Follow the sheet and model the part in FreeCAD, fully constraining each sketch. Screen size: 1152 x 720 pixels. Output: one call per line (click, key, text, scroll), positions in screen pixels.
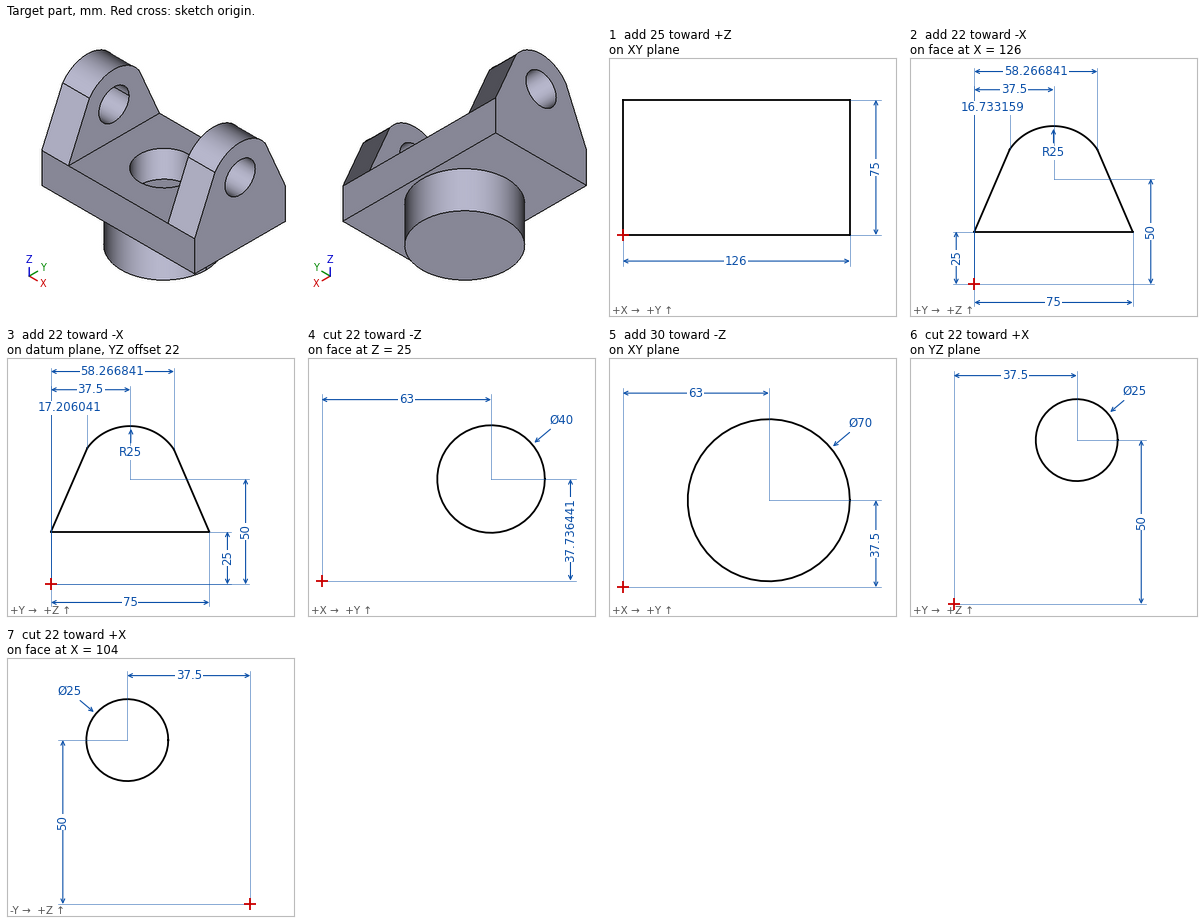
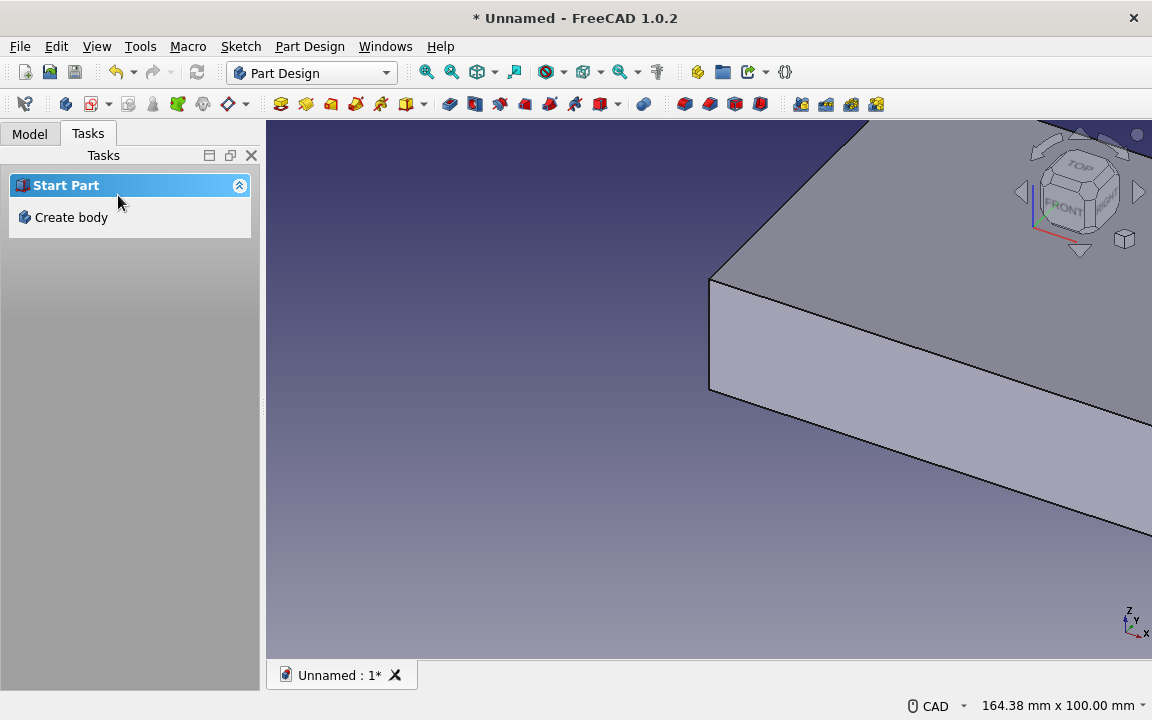
click(427, 72)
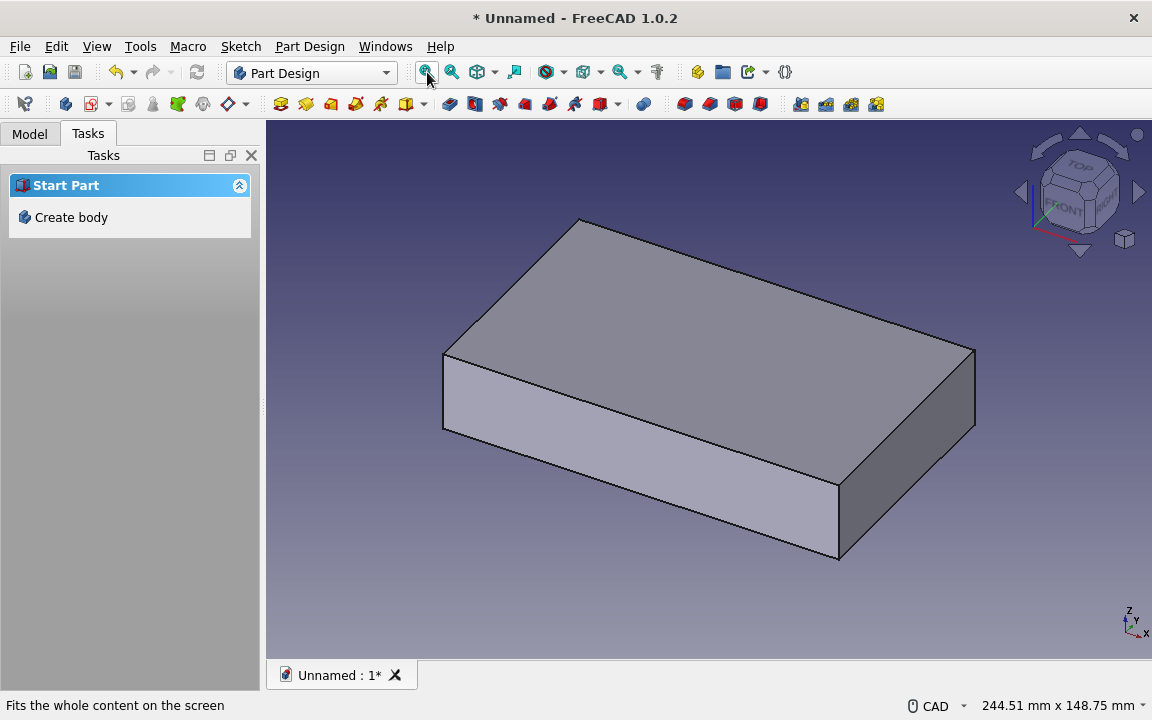
click(946, 415)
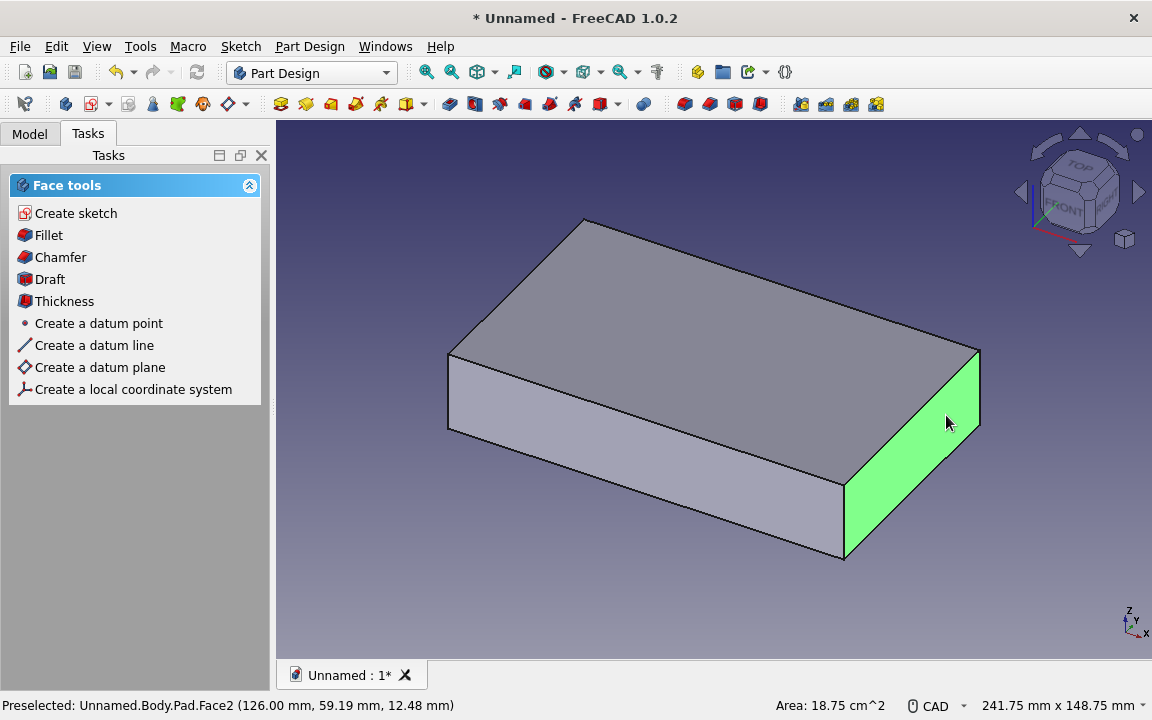
click(90, 104)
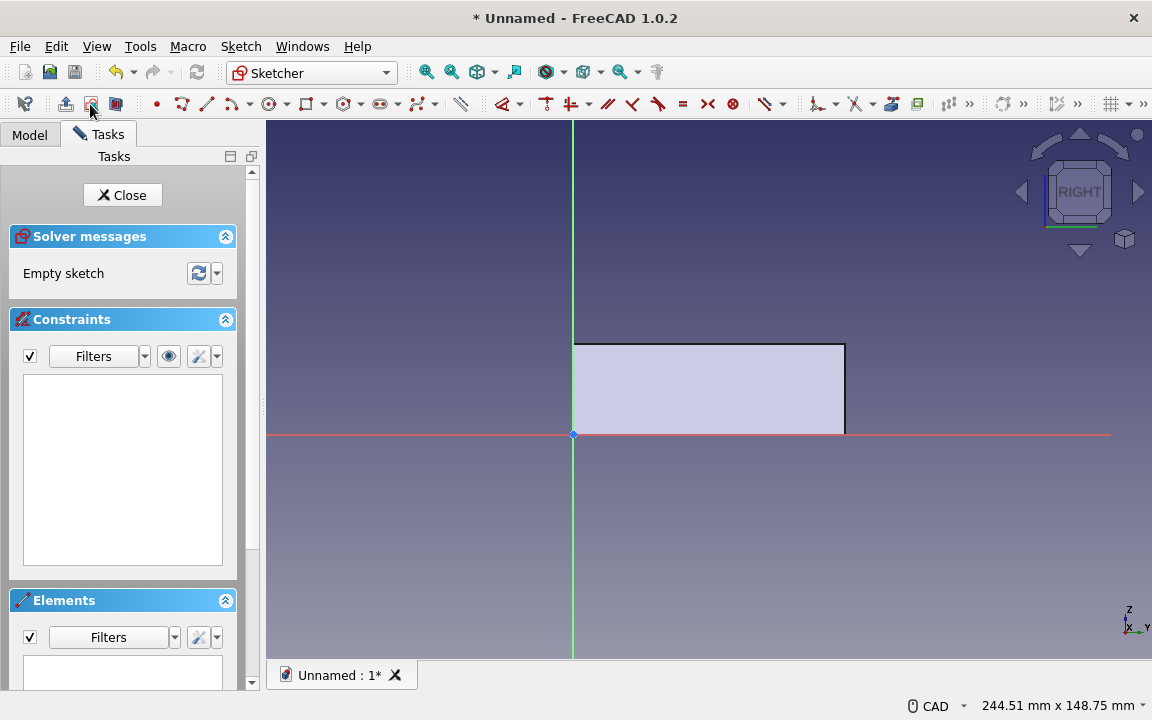
scroll(331, 631, down, 1)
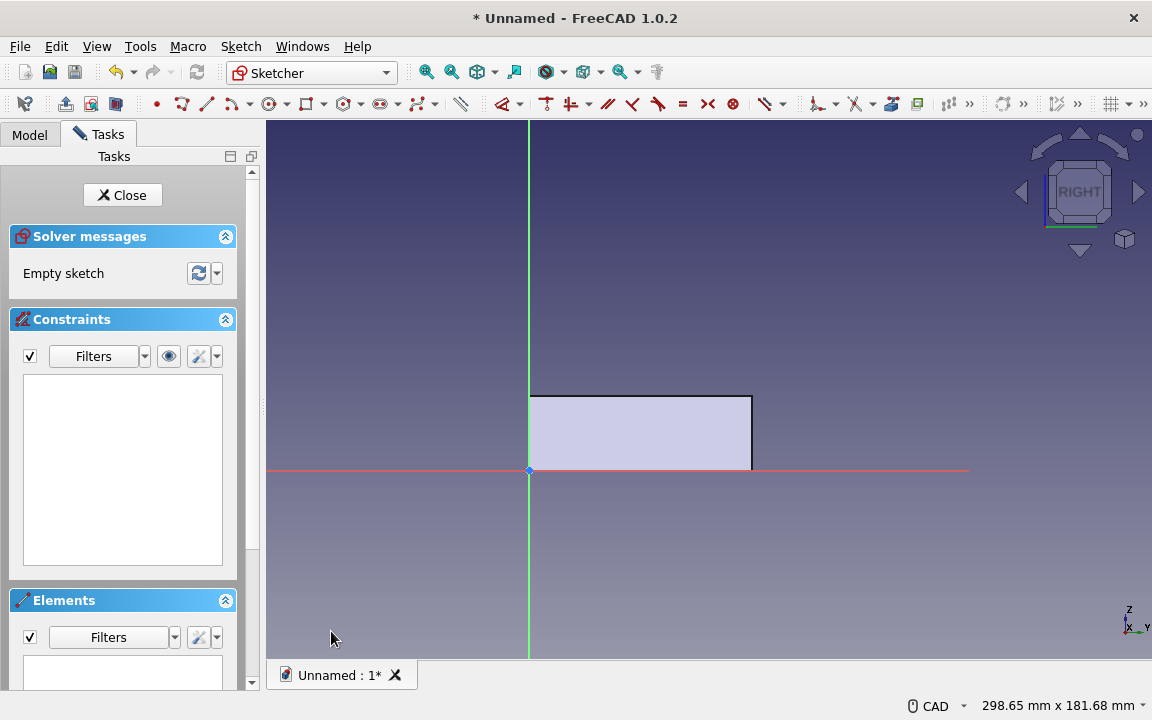
scroll(640, 298, up, 2)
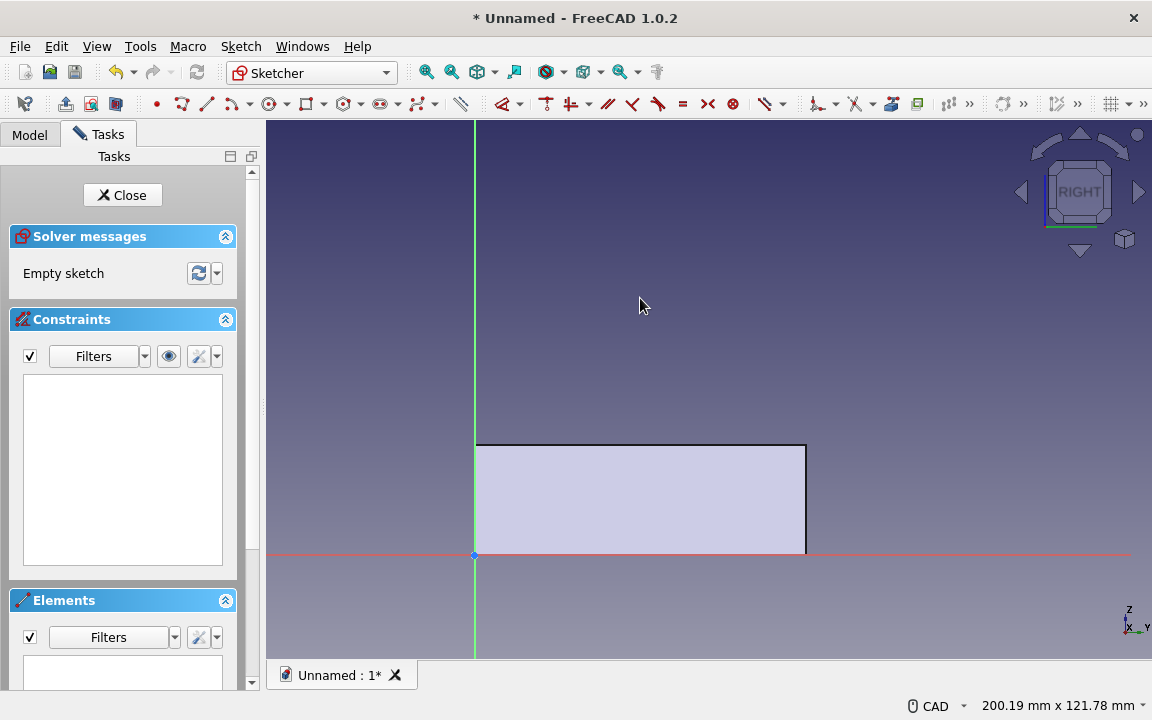
click(182, 104)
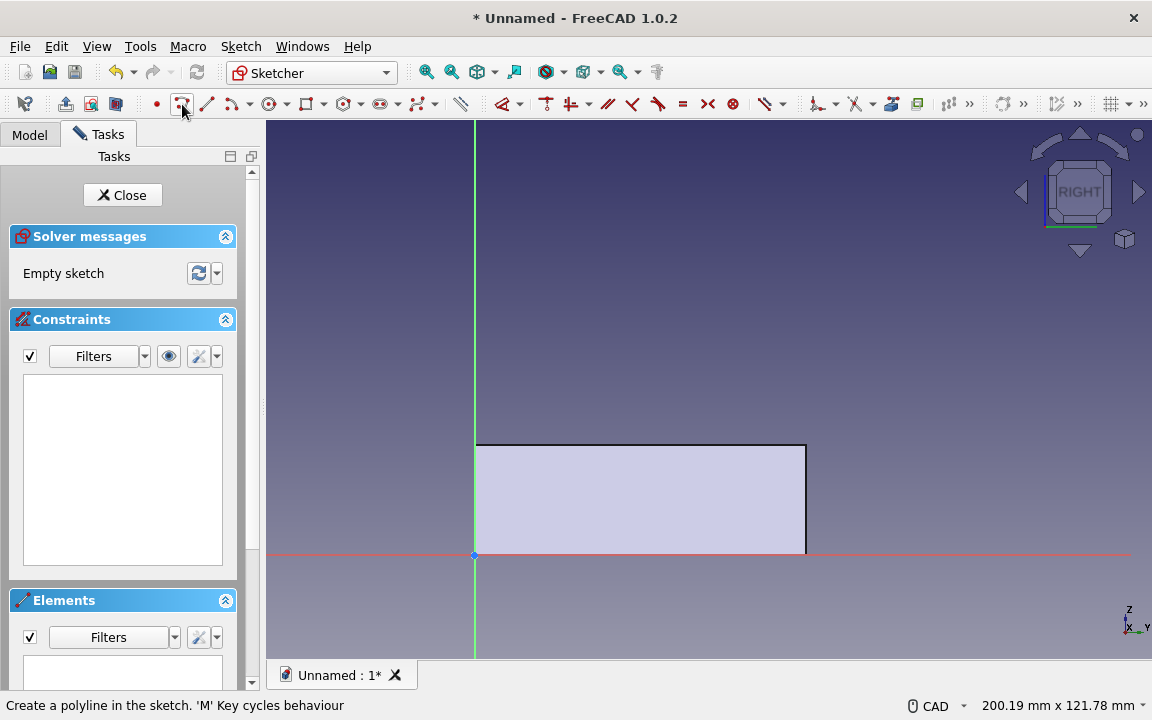
click(549, 272)
click(475, 445)
click(806, 445)
click(732, 272)
right_click(732, 272)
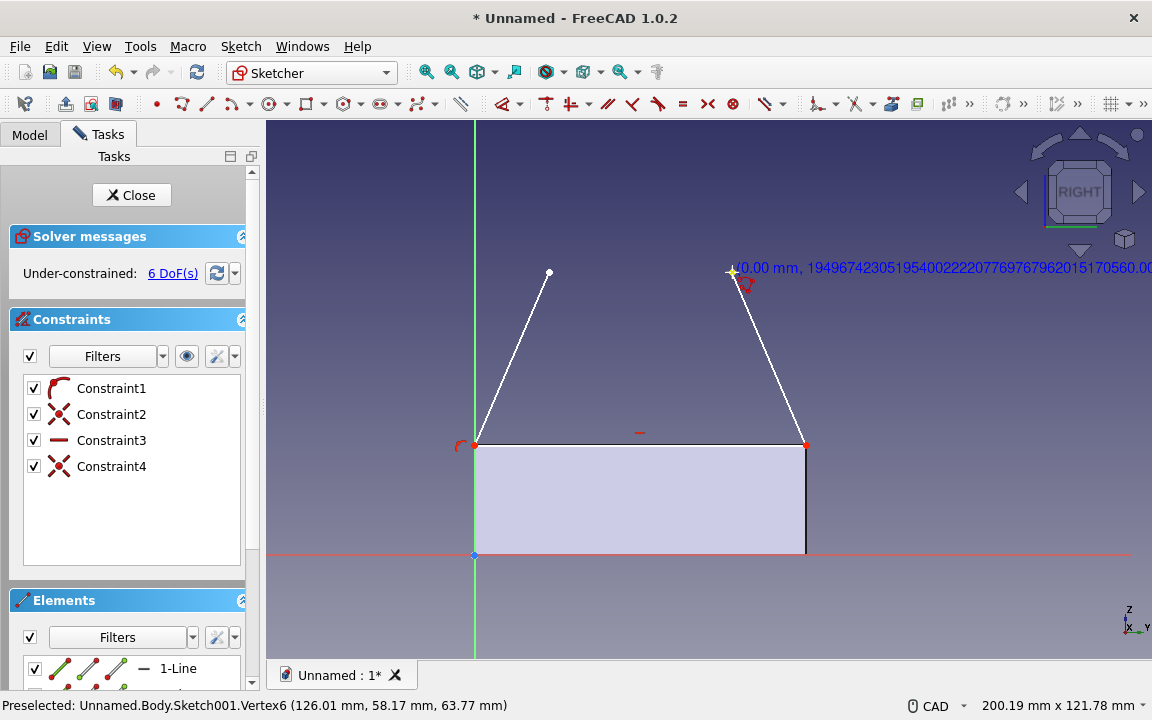
click(250, 104)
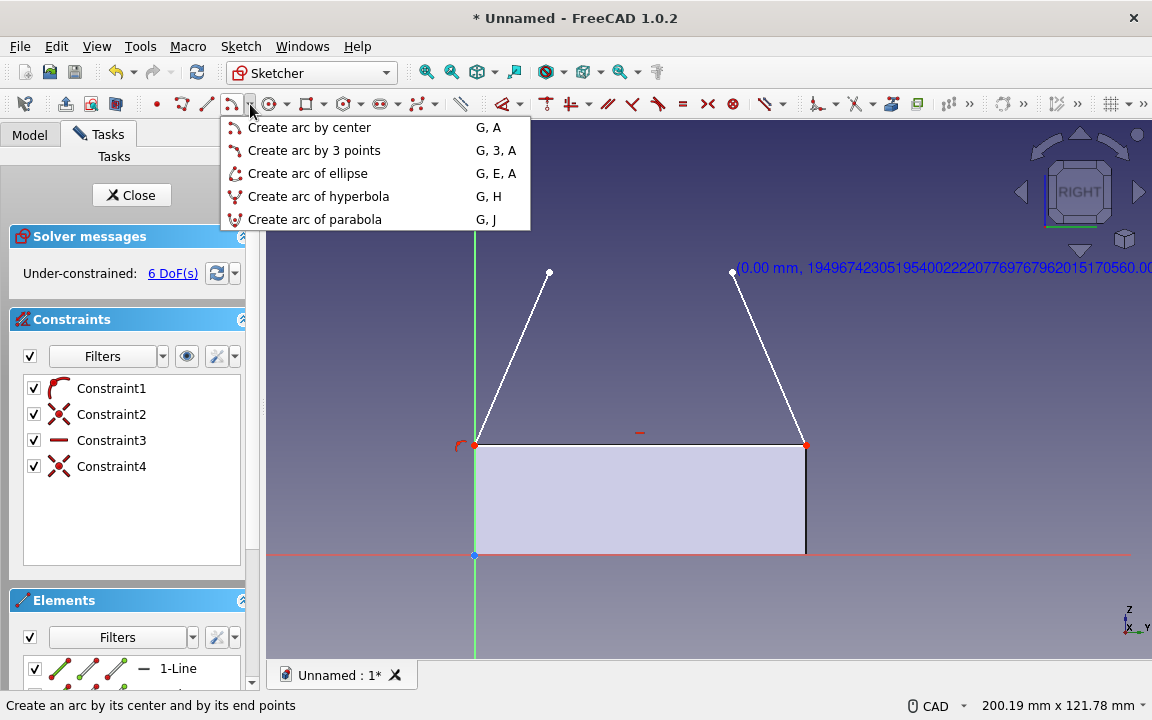
click(376, 150)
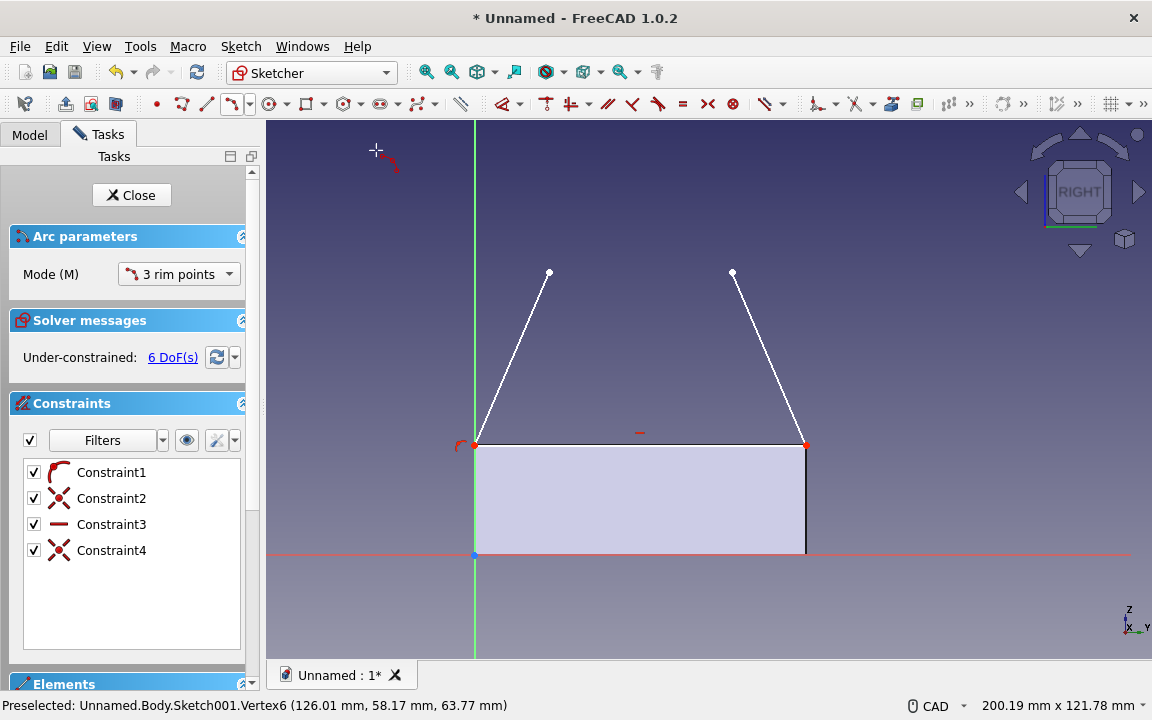
click(732, 273)
click(549, 273)
click(641, 223)
key(Escape)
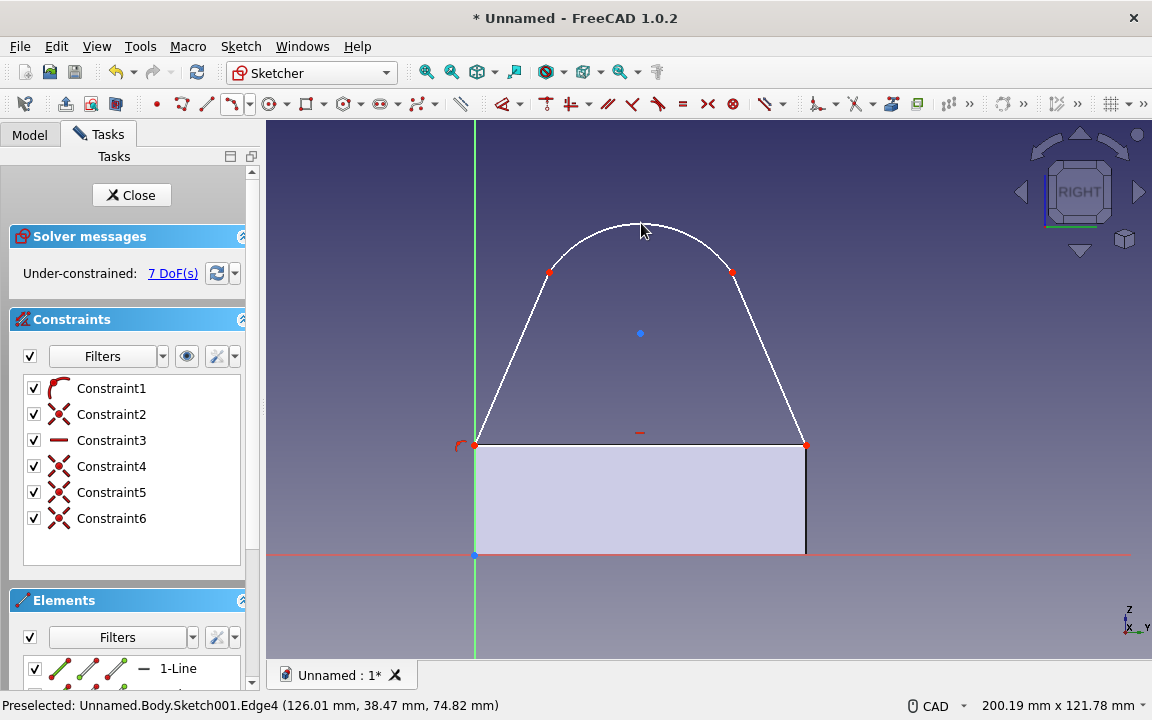
click(502, 104)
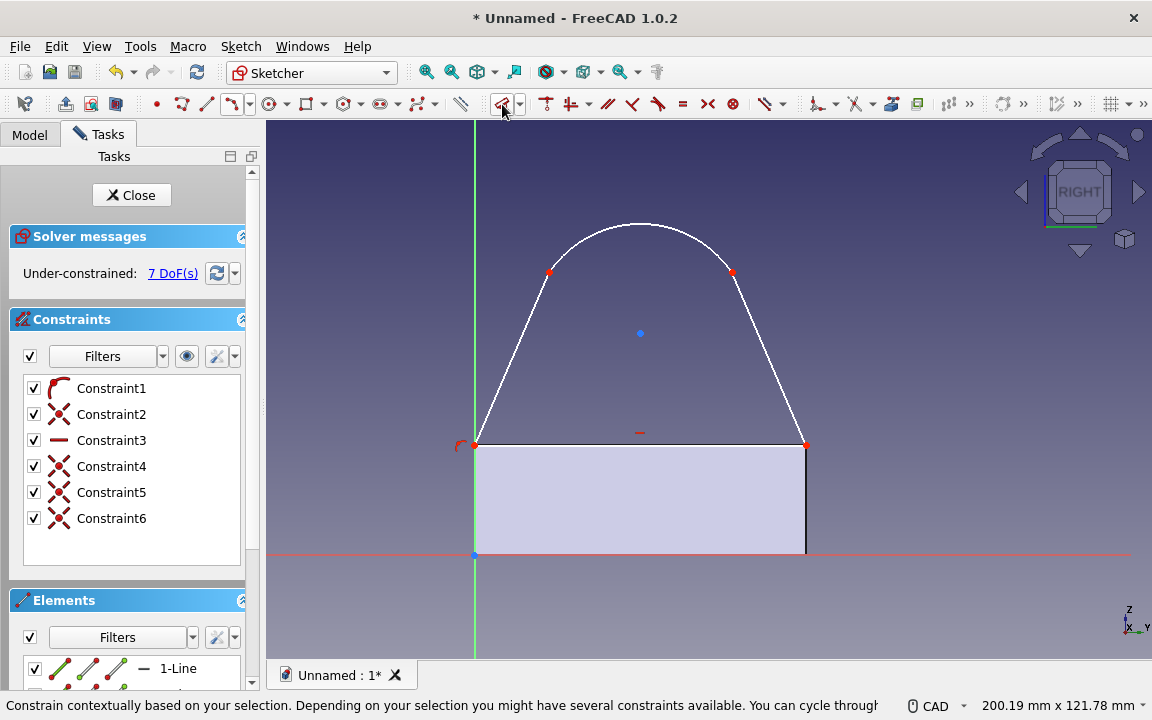
click(683, 232)
click(695, 202)